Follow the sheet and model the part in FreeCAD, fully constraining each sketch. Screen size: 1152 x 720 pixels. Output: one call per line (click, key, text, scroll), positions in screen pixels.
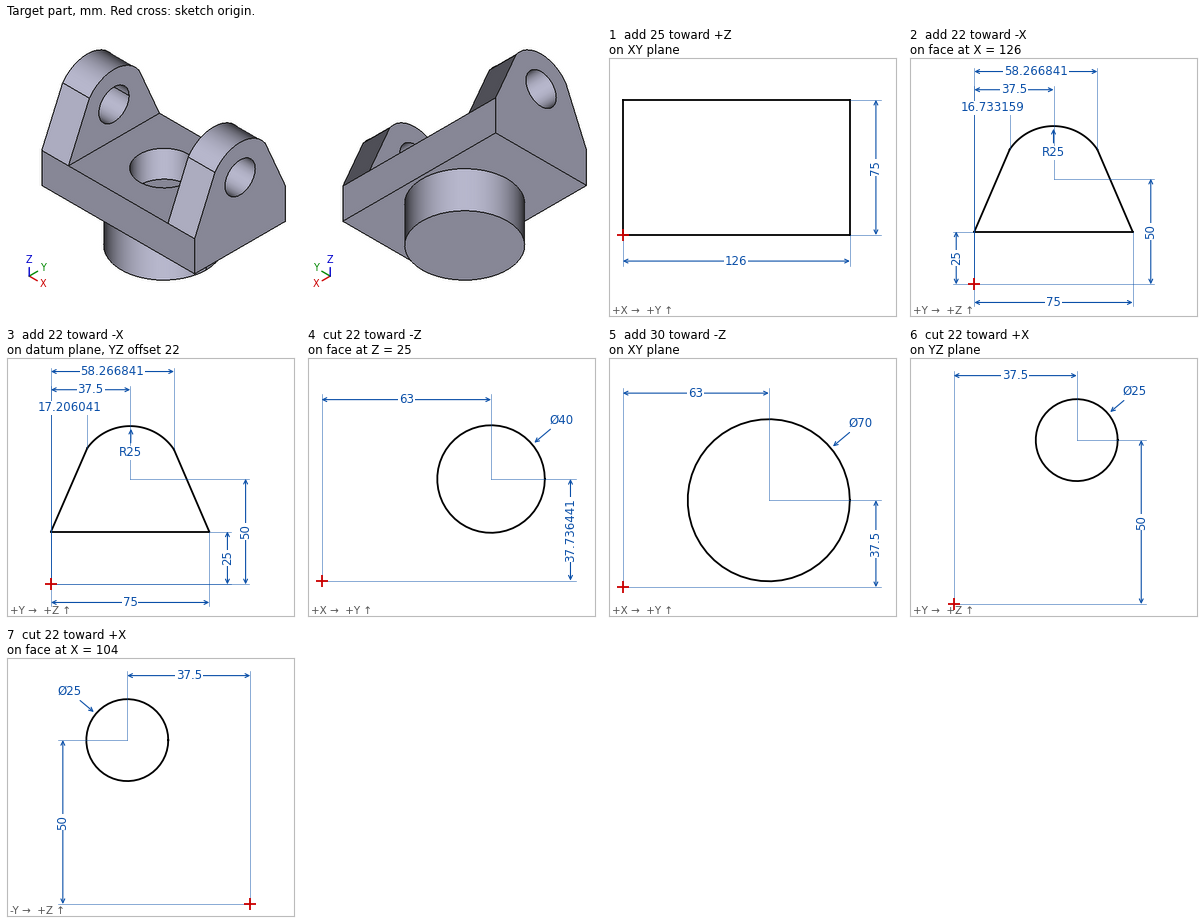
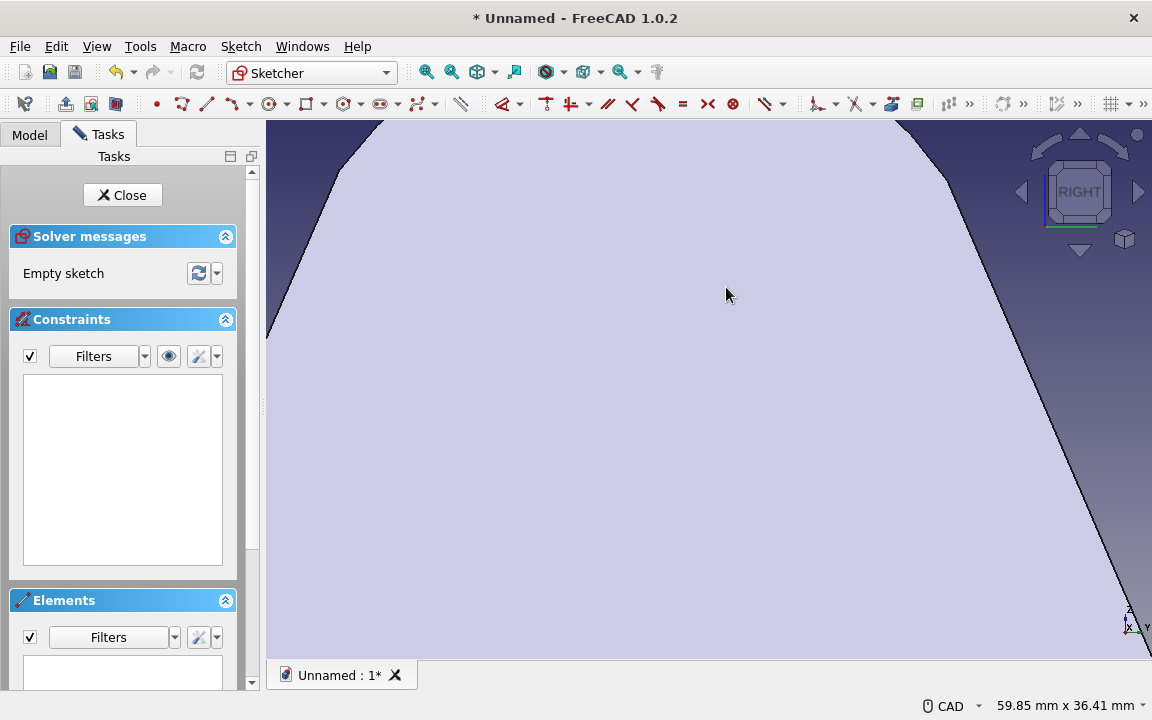
click(268, 104)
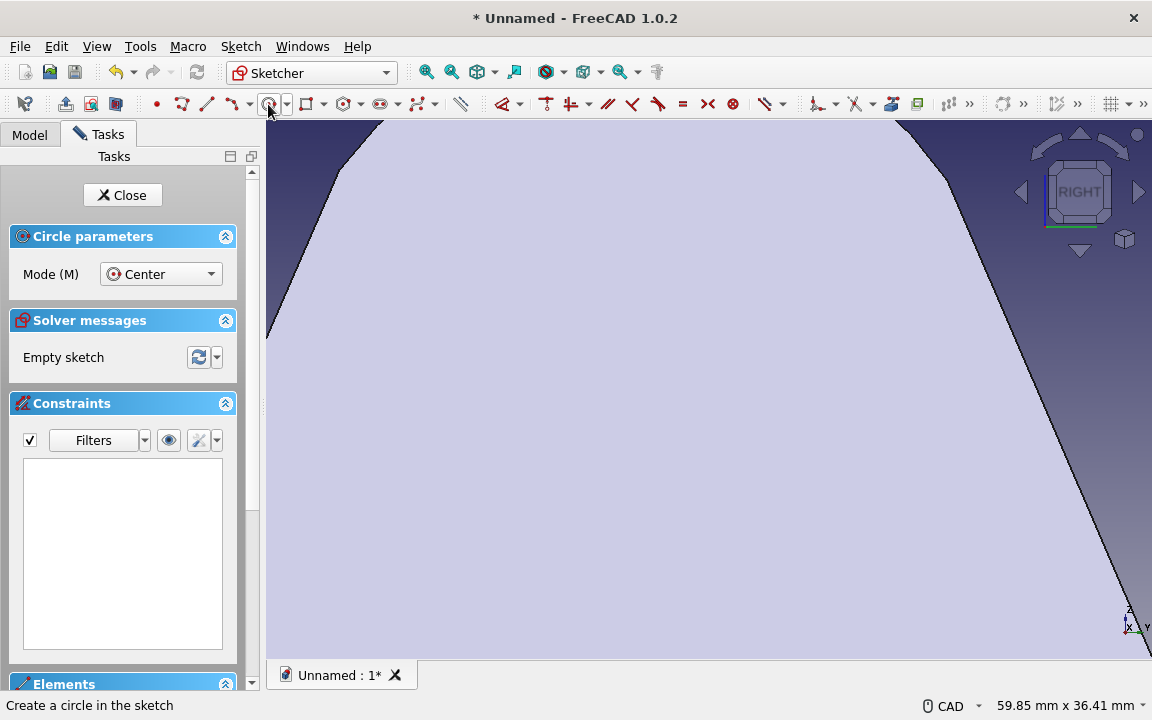
click(640, 386)
move(771, 256)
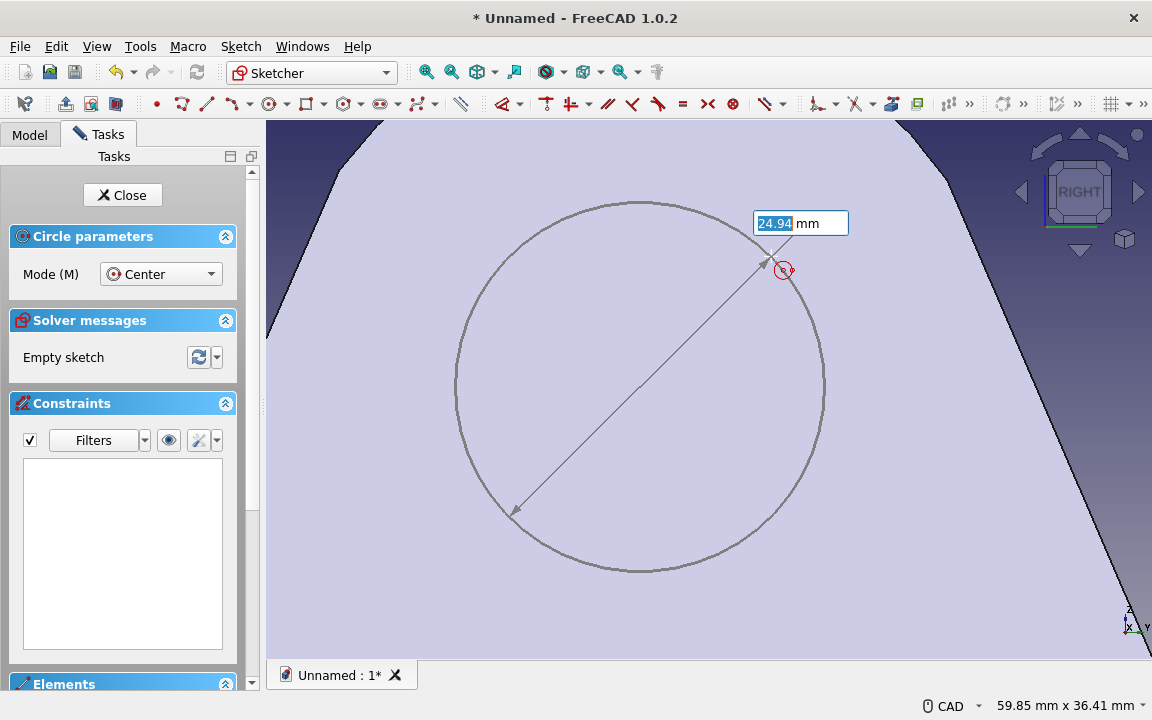
text(25)
key(Return)
key(Escape)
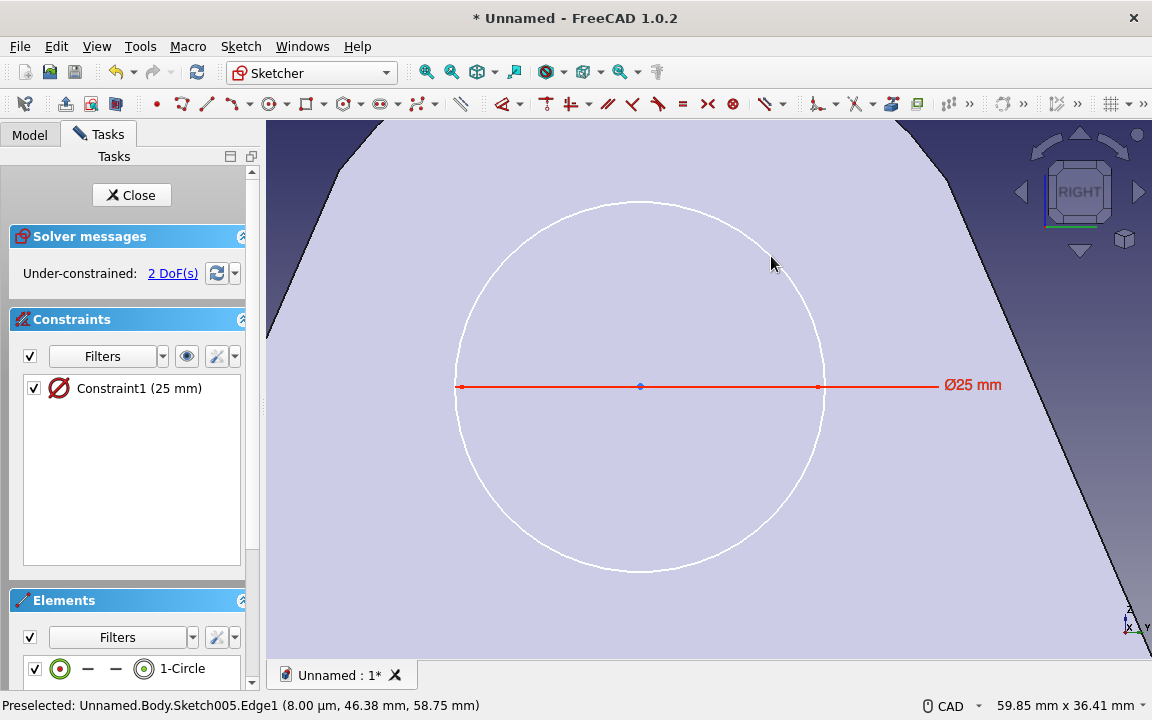
click(502, 104)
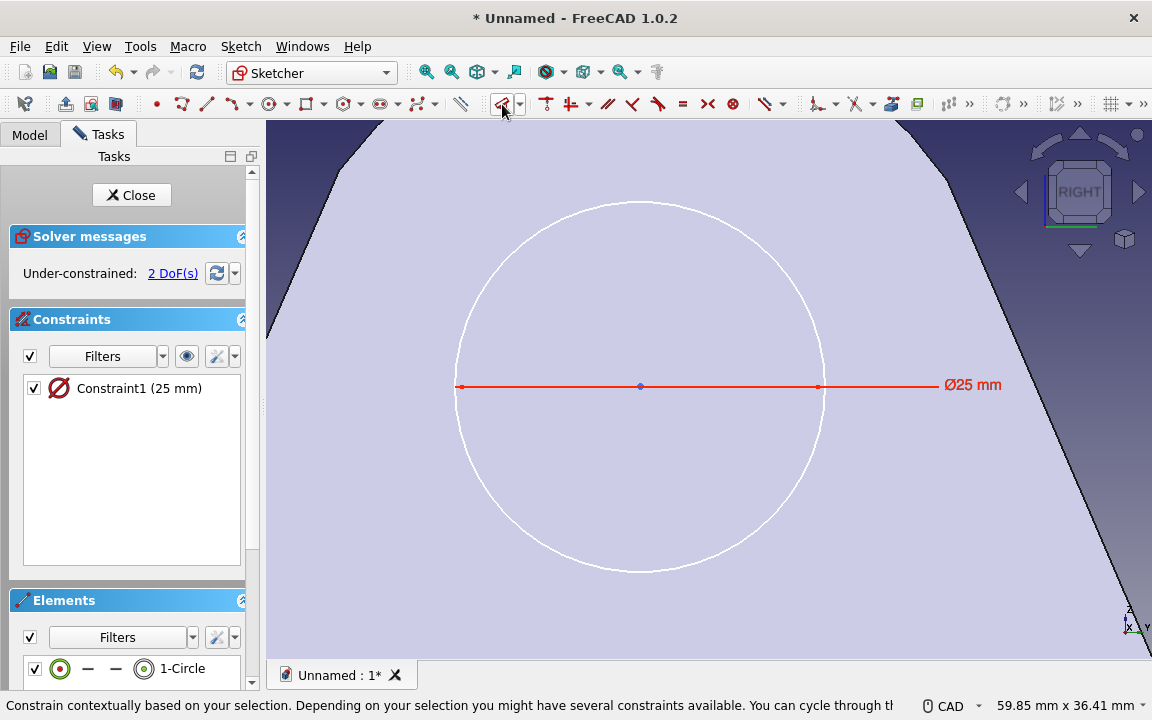
click(640, 387)
click(674, 509)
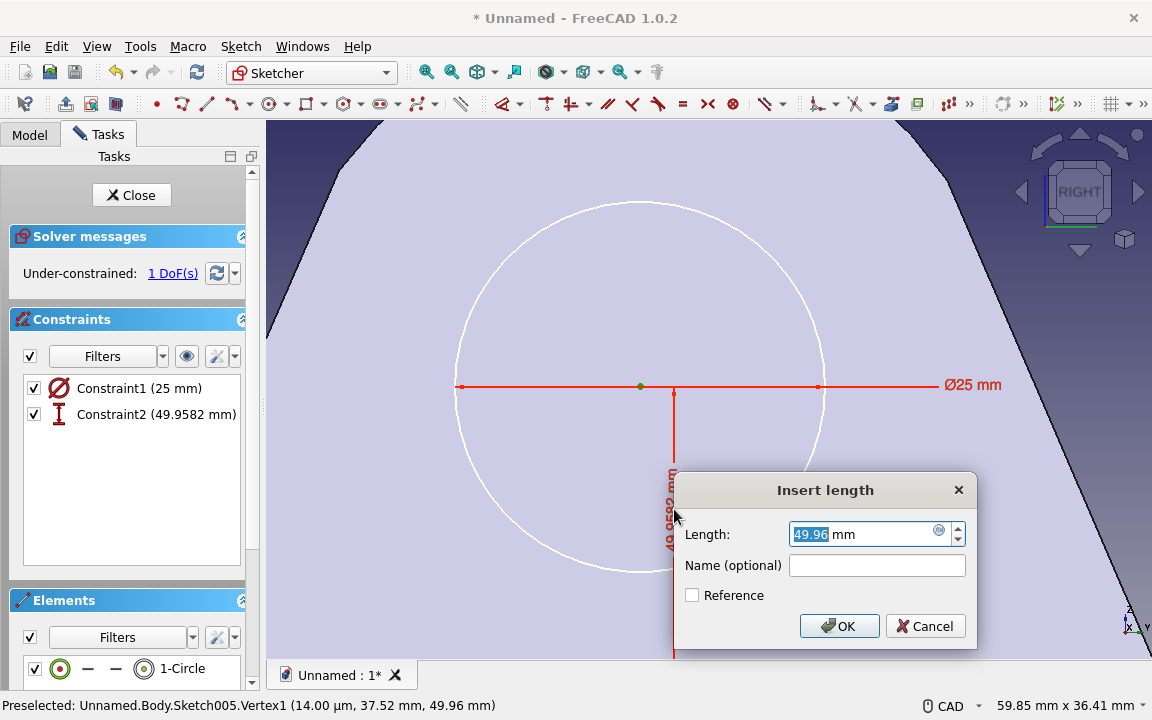
text(50)
key(Return)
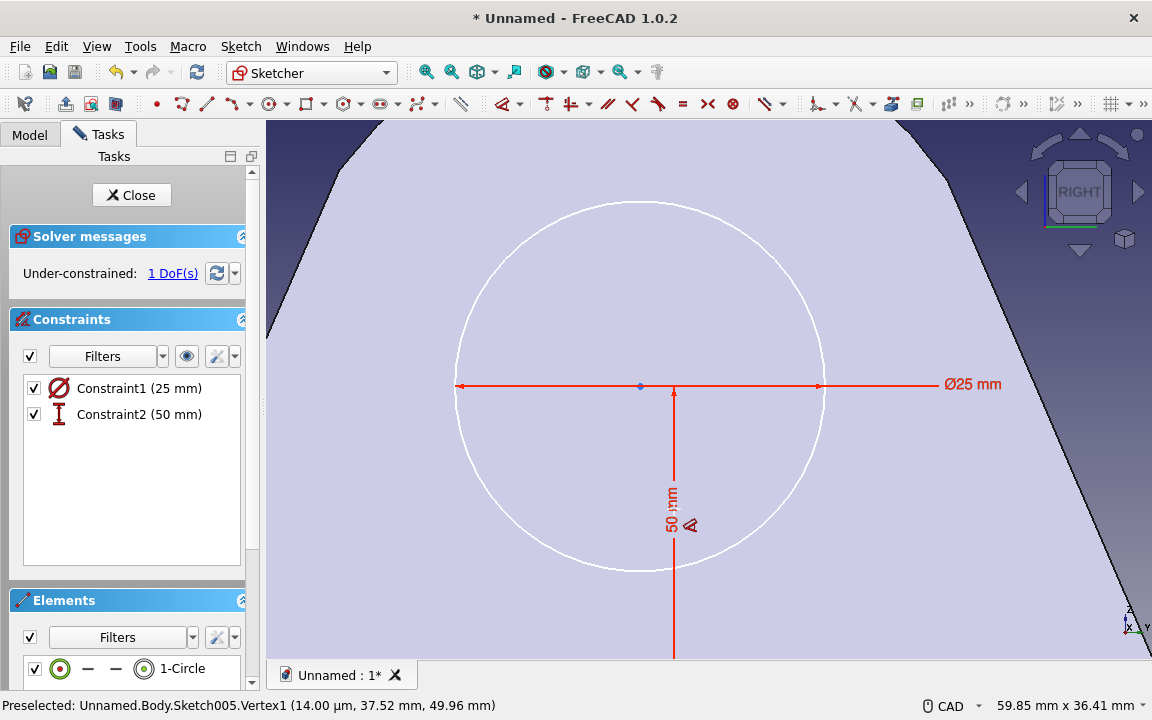
click(640, 386)
click(387, 352)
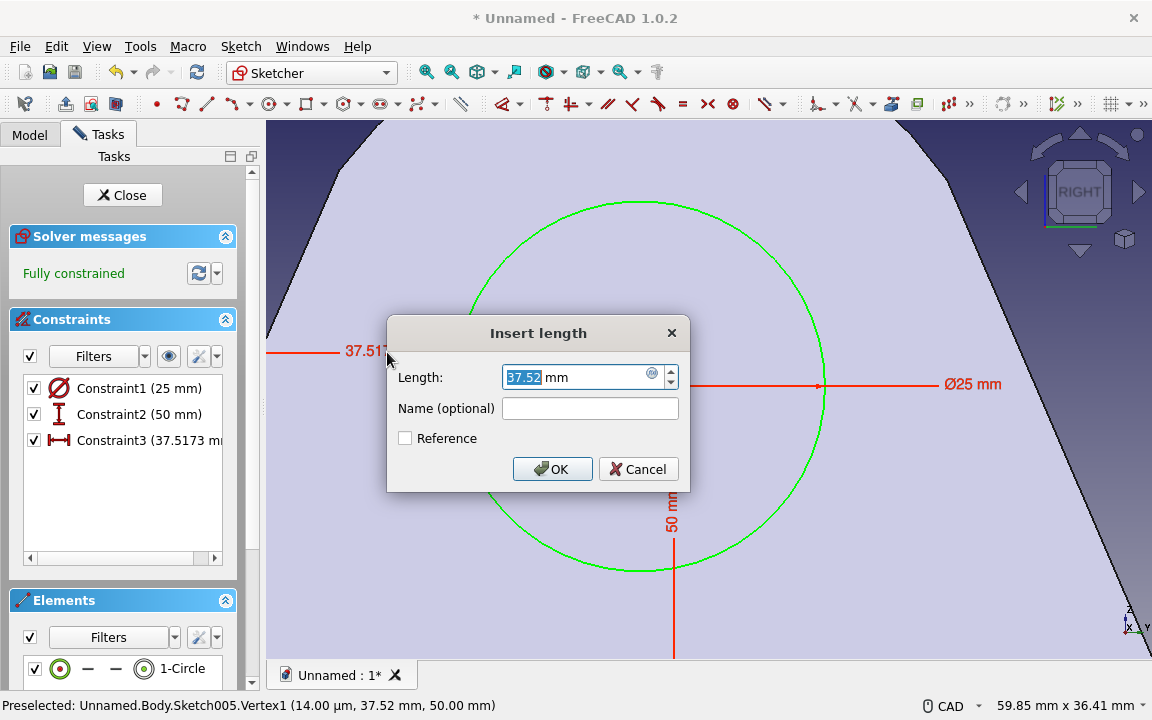
text(37.5)
key(Return)
key(Escape)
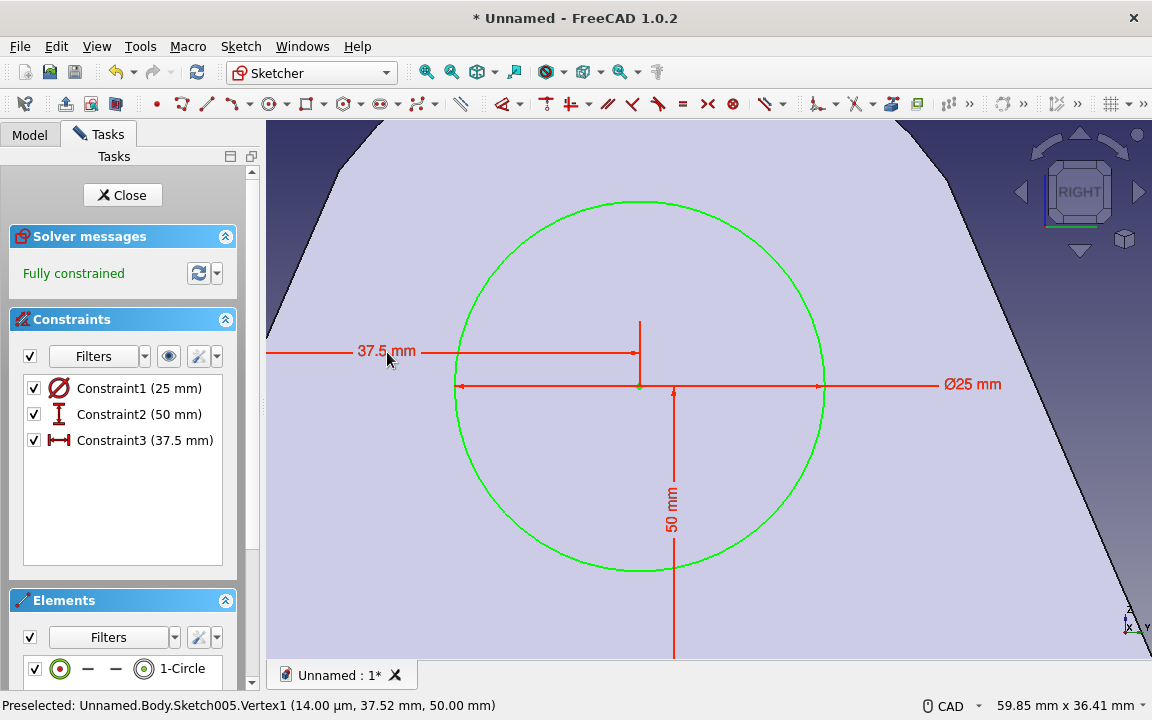
click(123, 195)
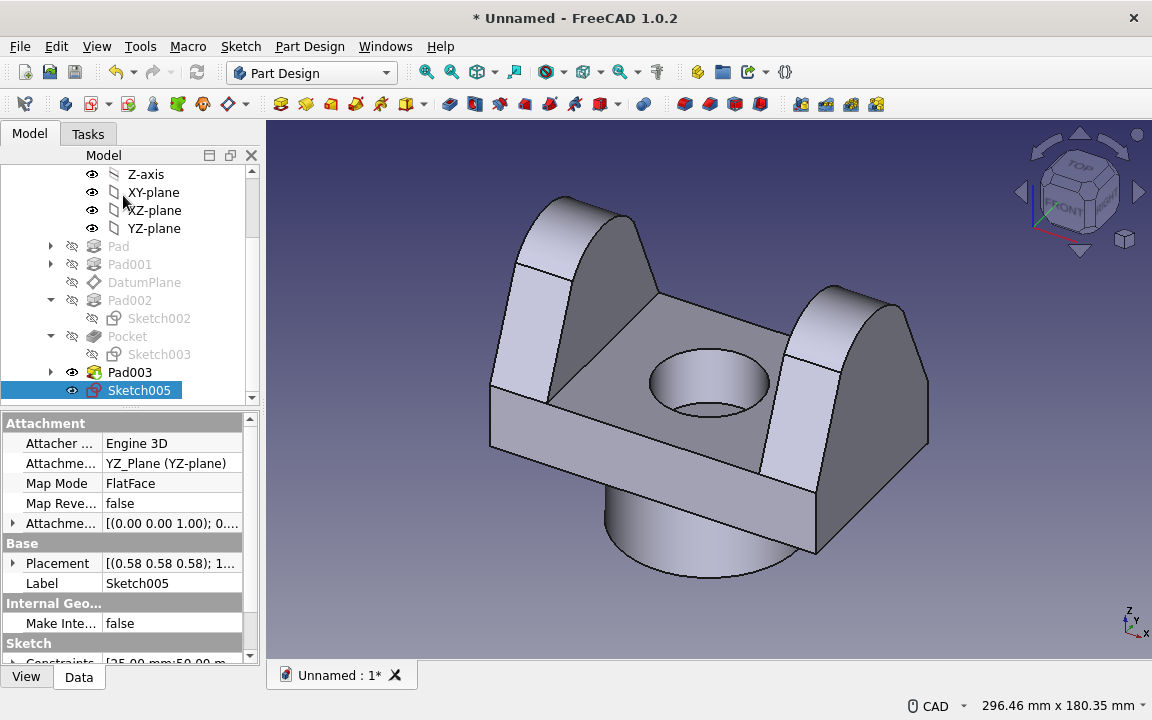
click(450, 104)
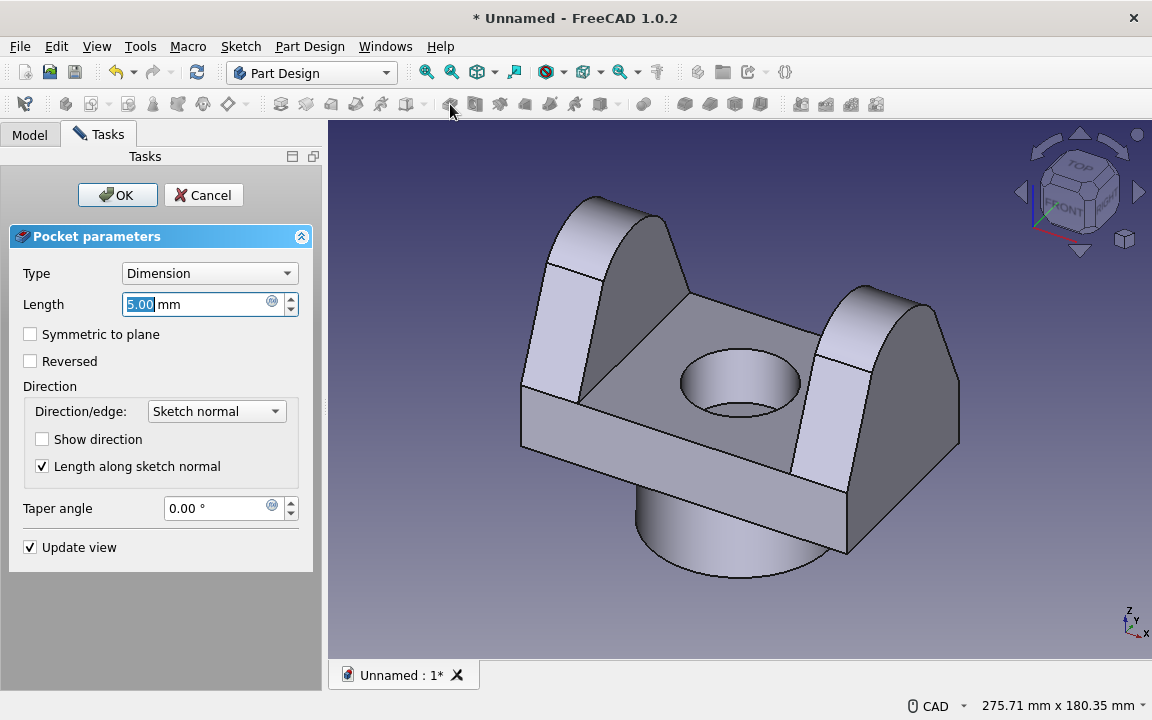
text(22)
key(Tab)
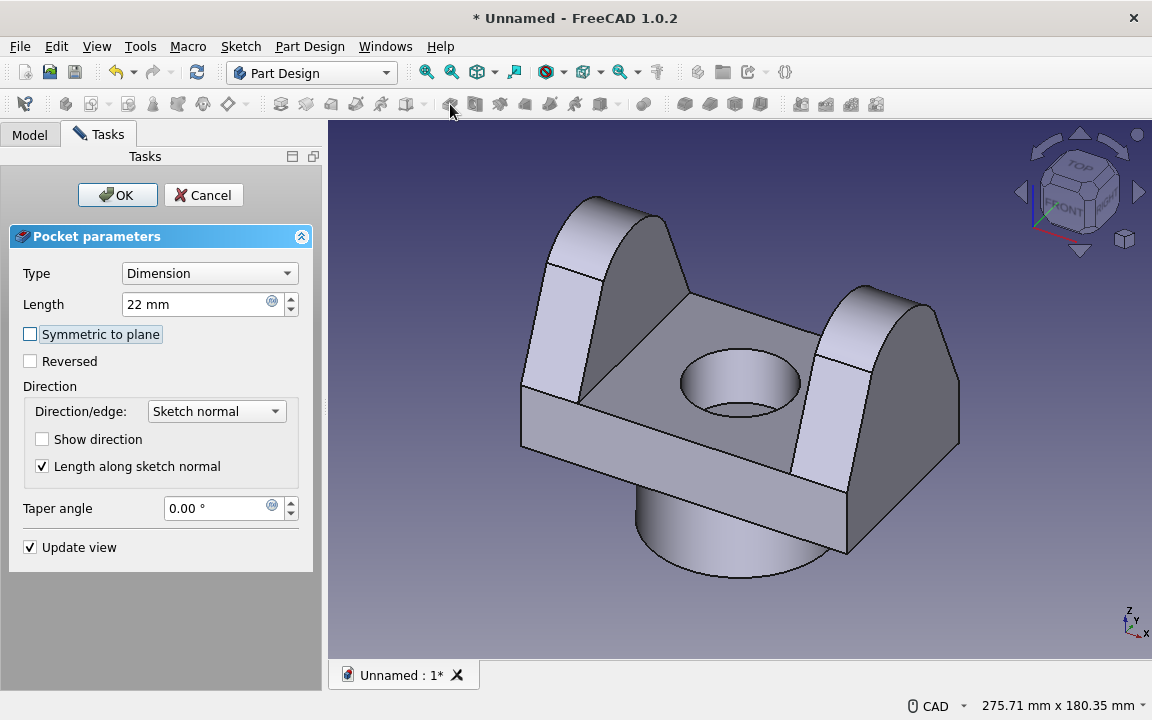
click(31, 361)